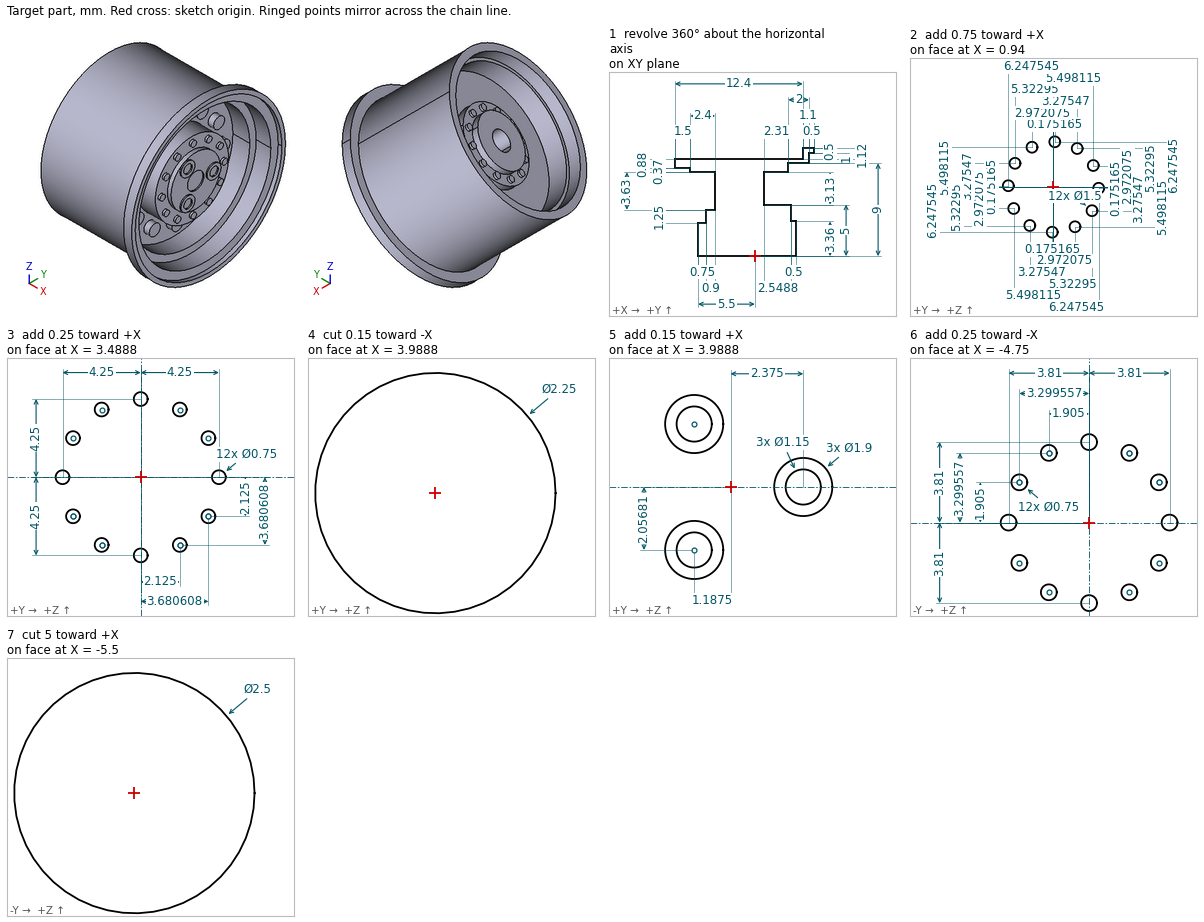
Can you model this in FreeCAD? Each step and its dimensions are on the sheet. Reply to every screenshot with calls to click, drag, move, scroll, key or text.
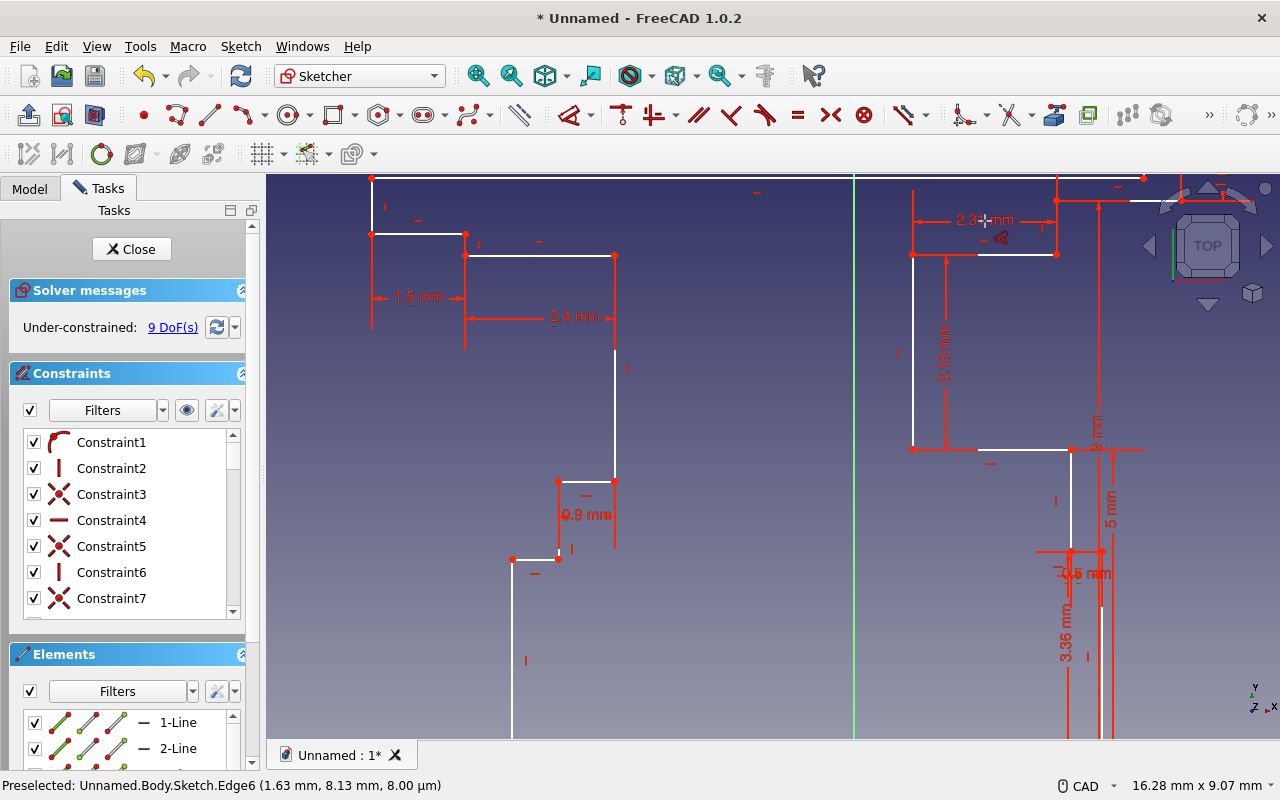
scroll(598, 484, down, 3)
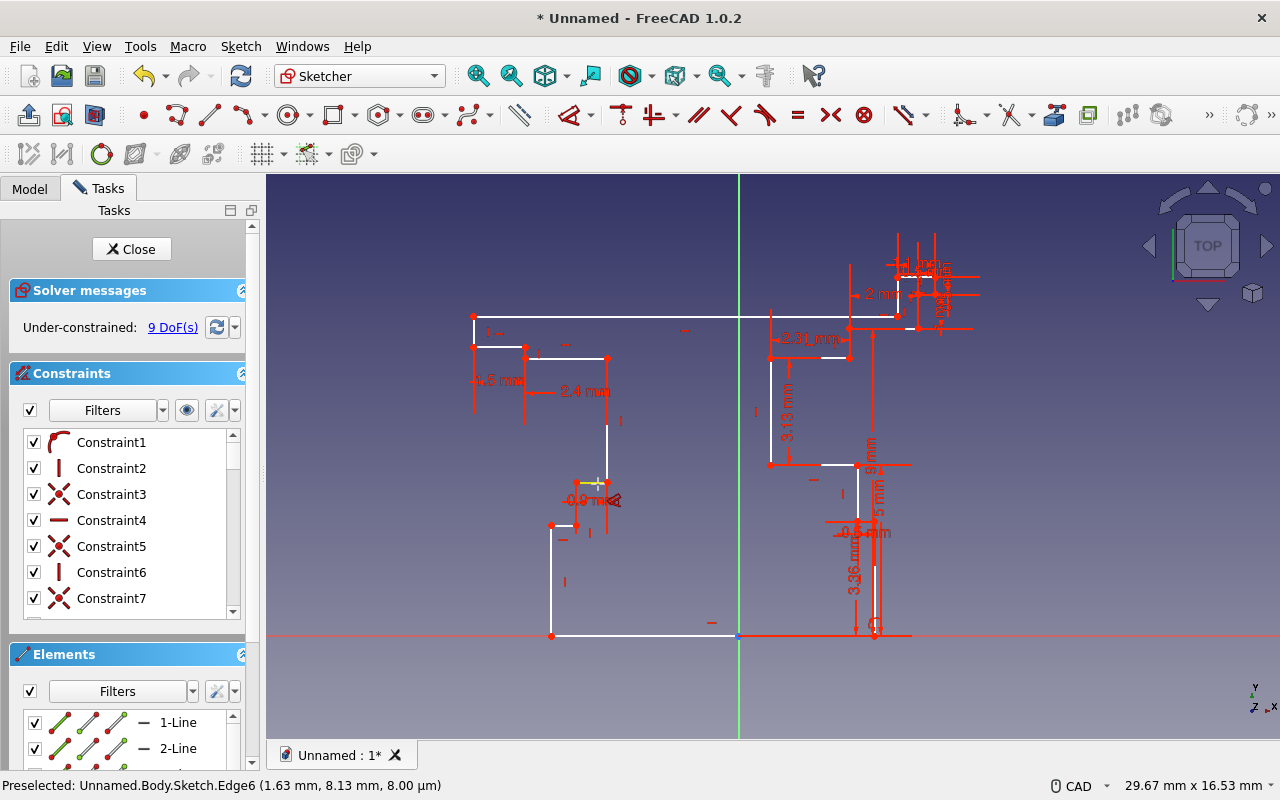
click(898, 289)
click(792, 297)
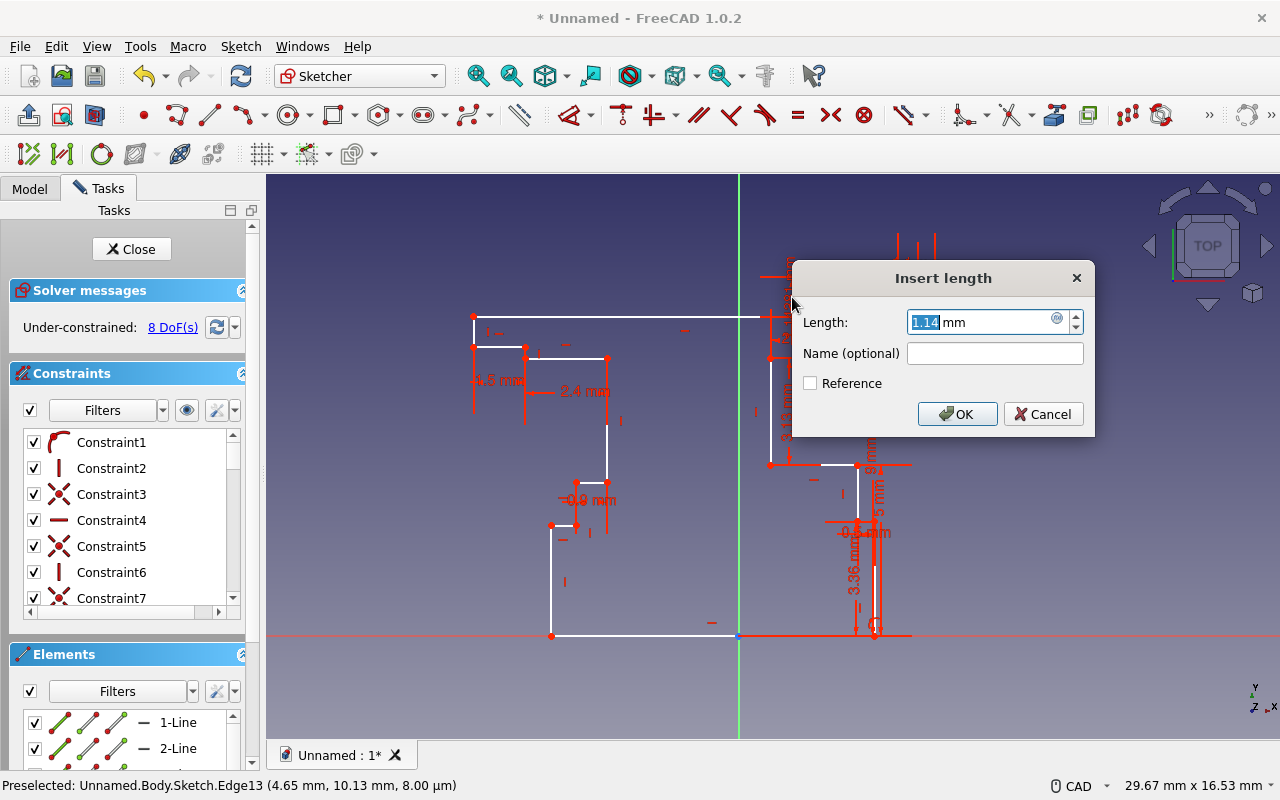
text(1.12)
key(Return)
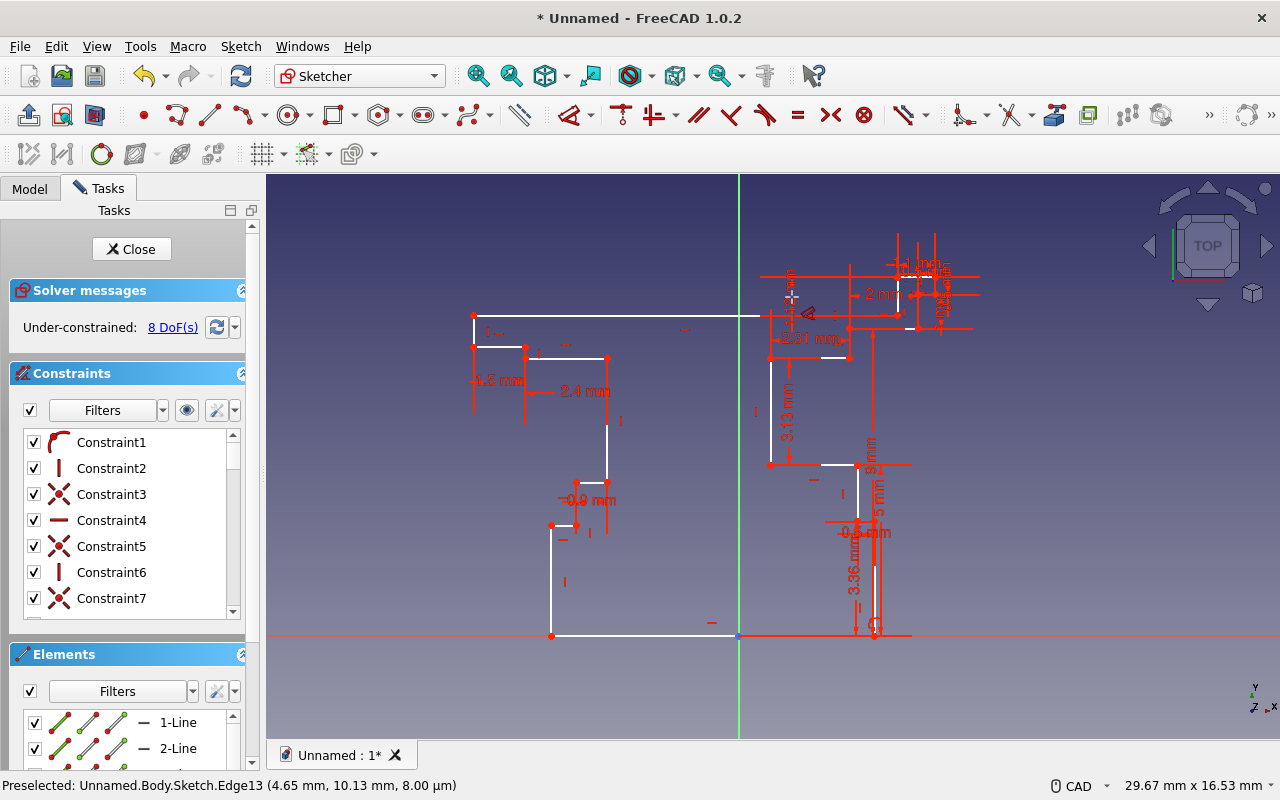
click(771, 316)
click(686, 282)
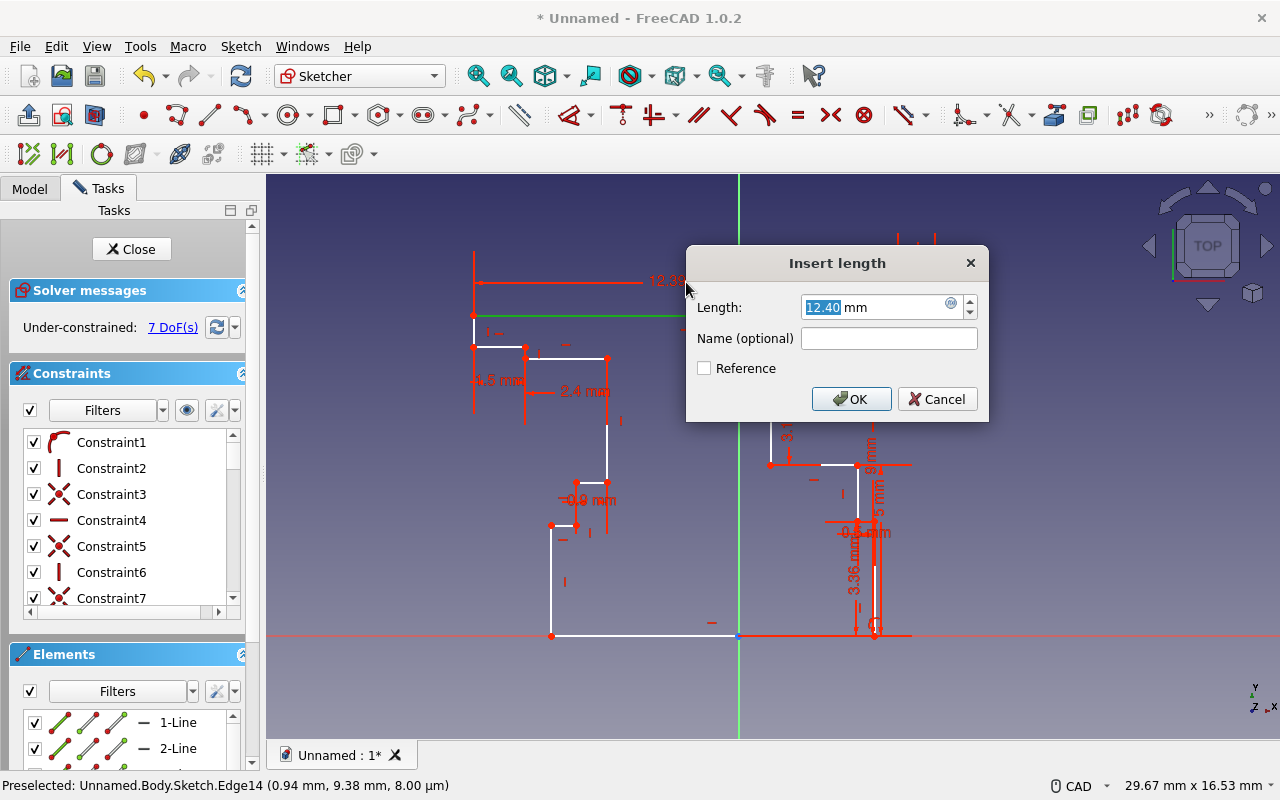
text(12.4)
key(Return)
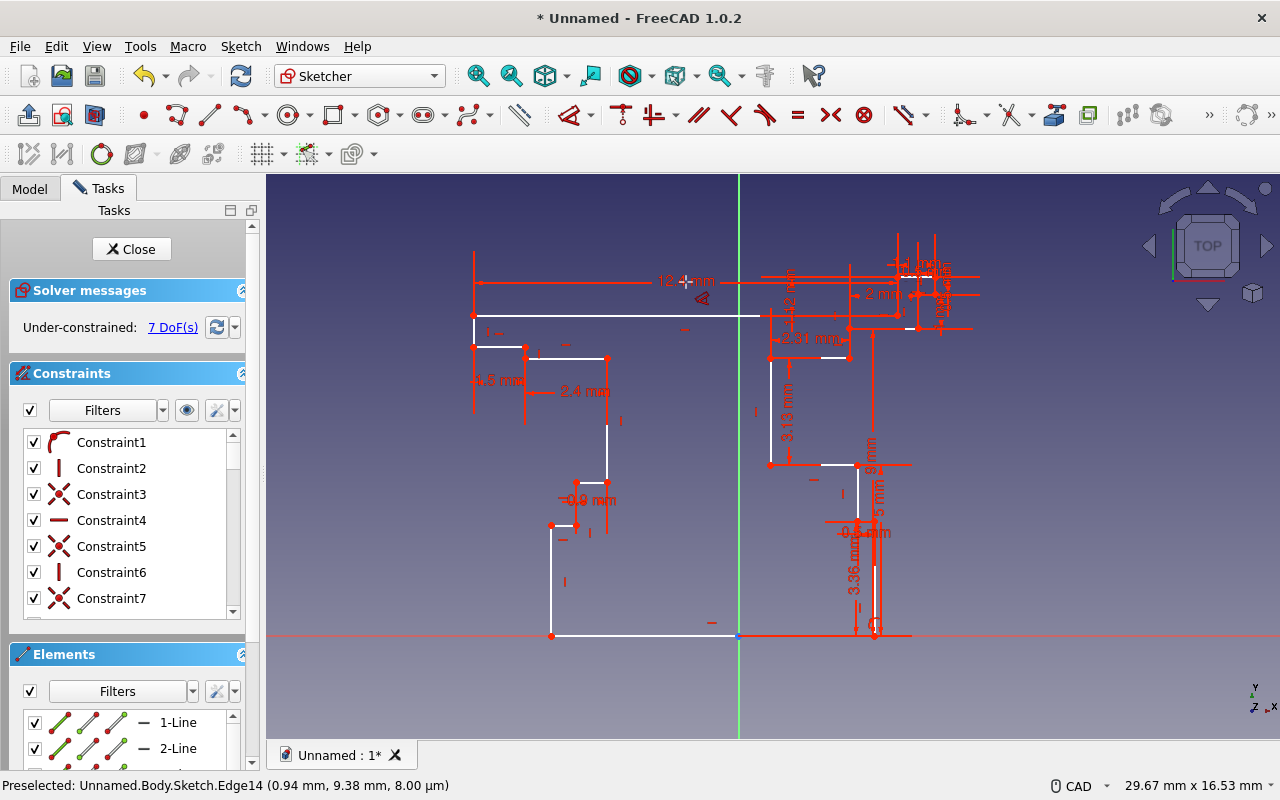
scroll(474, 325, up, 2)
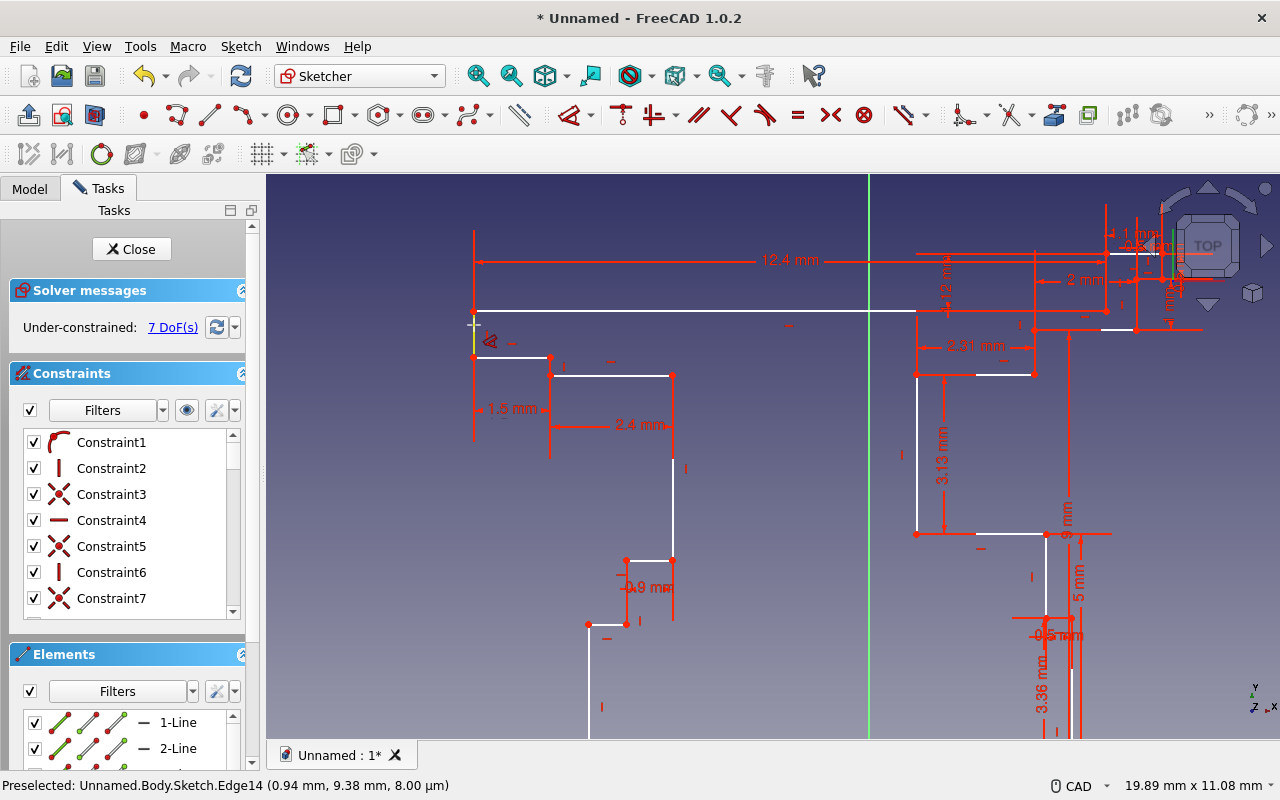
click(474, 325)
click(440, 335)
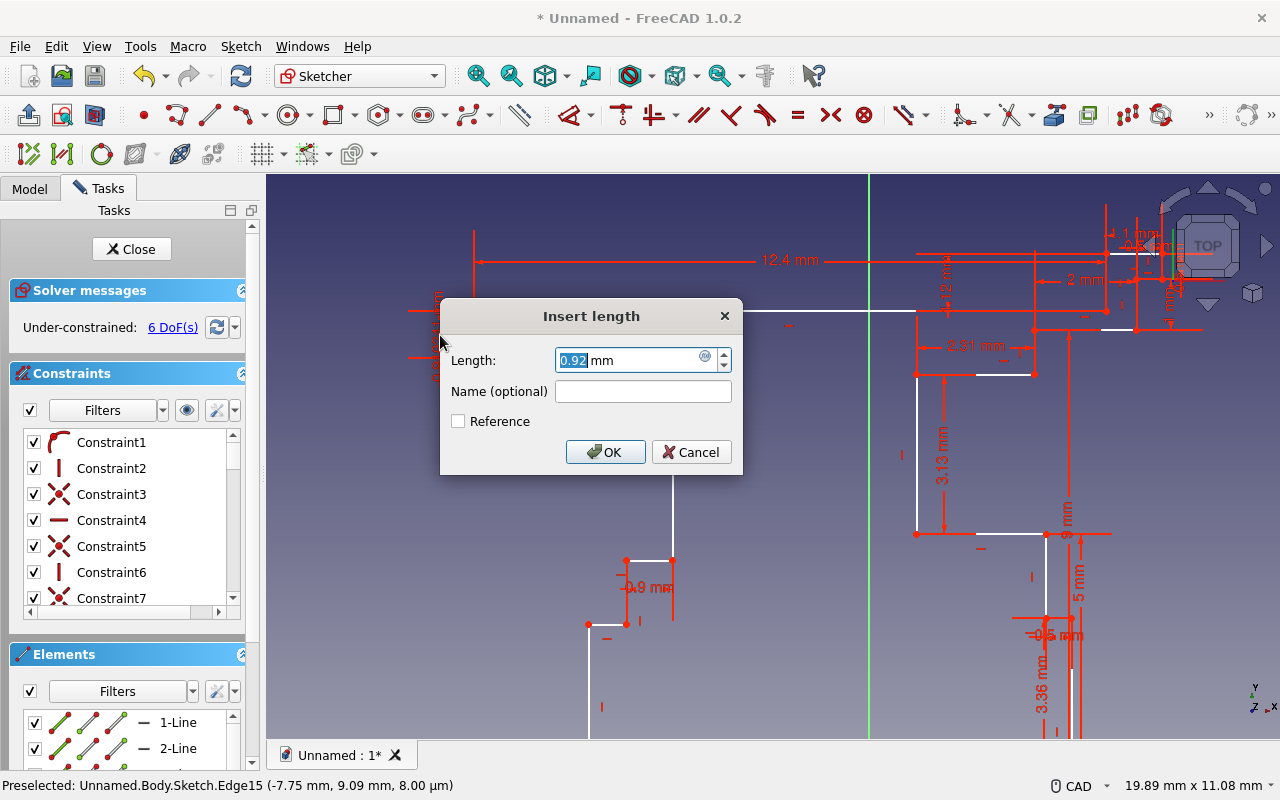
text(0.88)
key(Return)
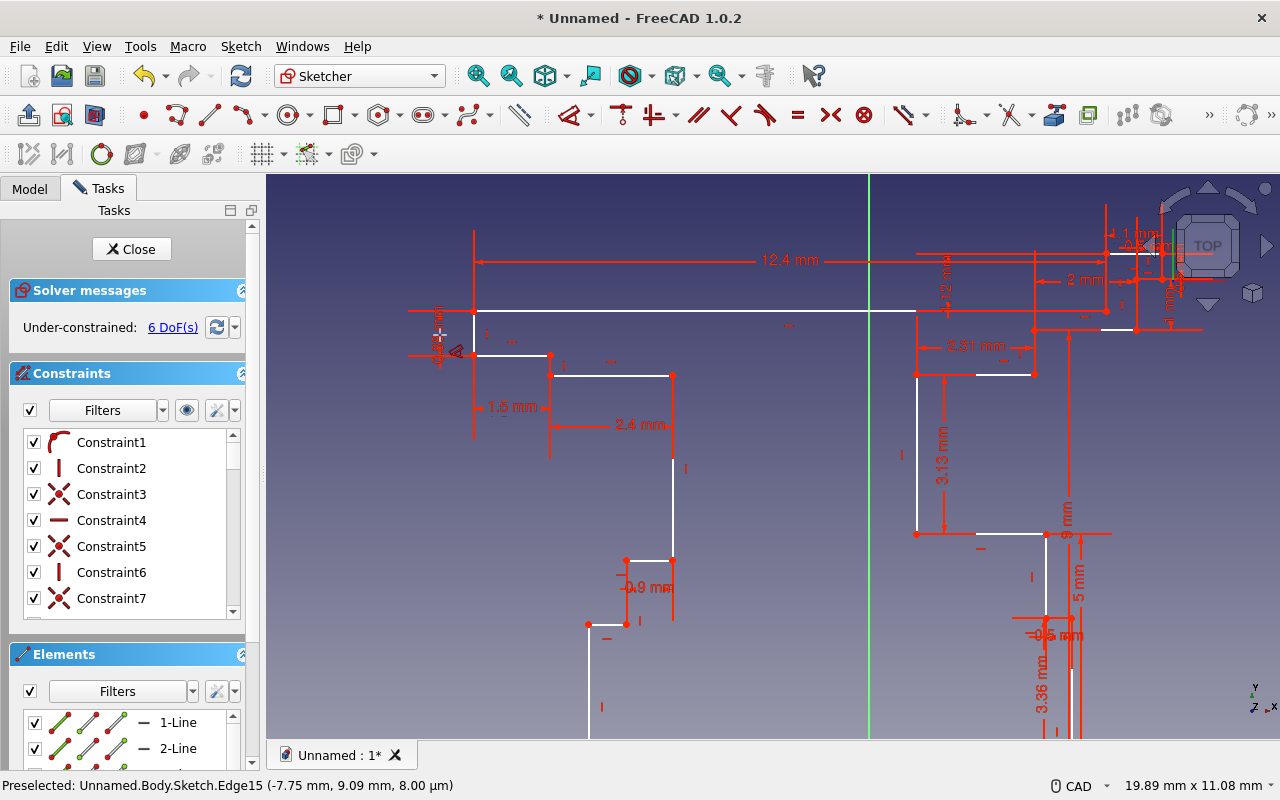
scroll(550, 366, up, 4)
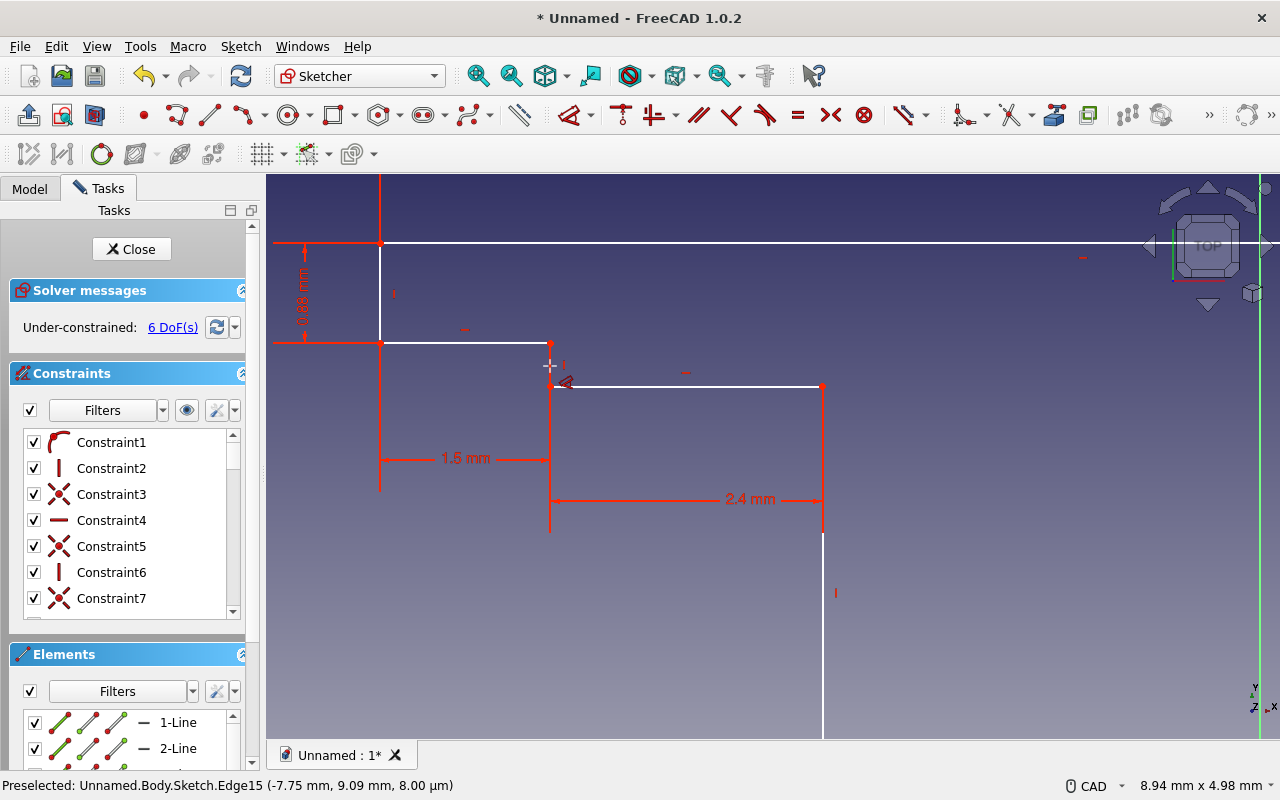
click(550, 365)
click(516, 365)